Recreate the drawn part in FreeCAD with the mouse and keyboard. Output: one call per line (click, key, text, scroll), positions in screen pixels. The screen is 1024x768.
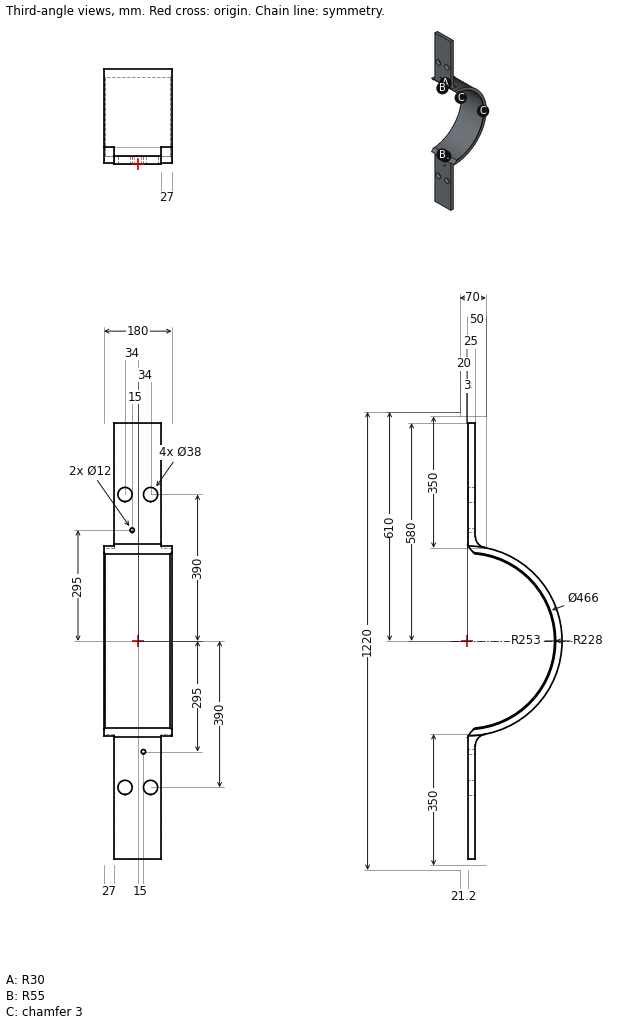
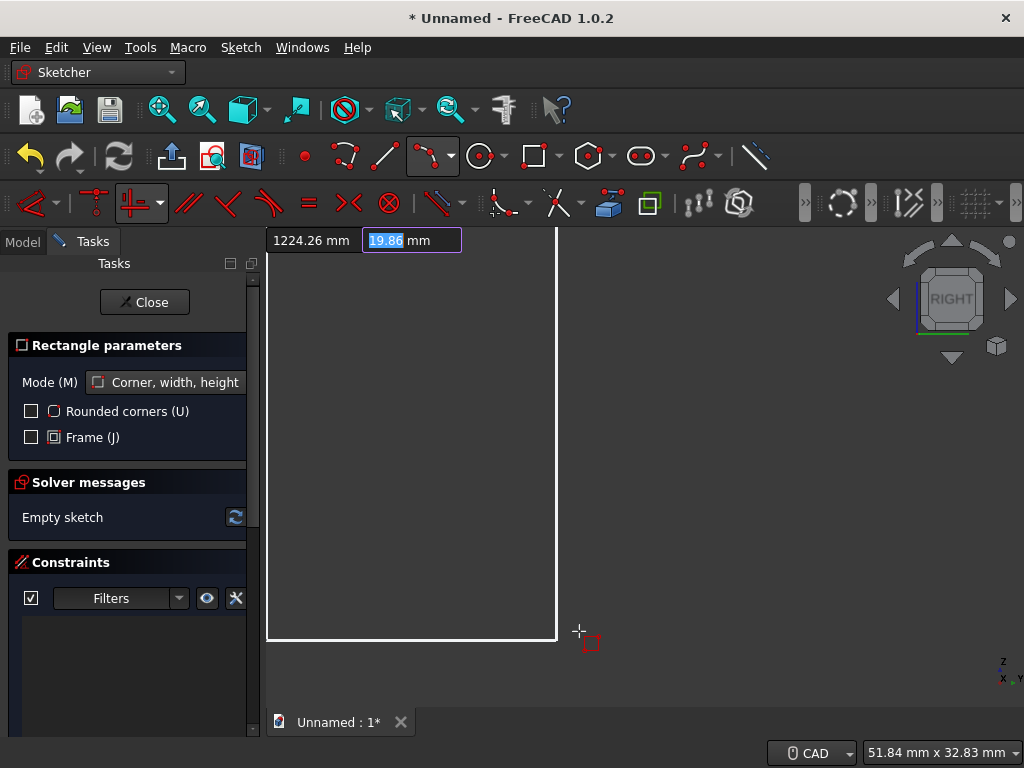
click(579, 561)
key(Escape)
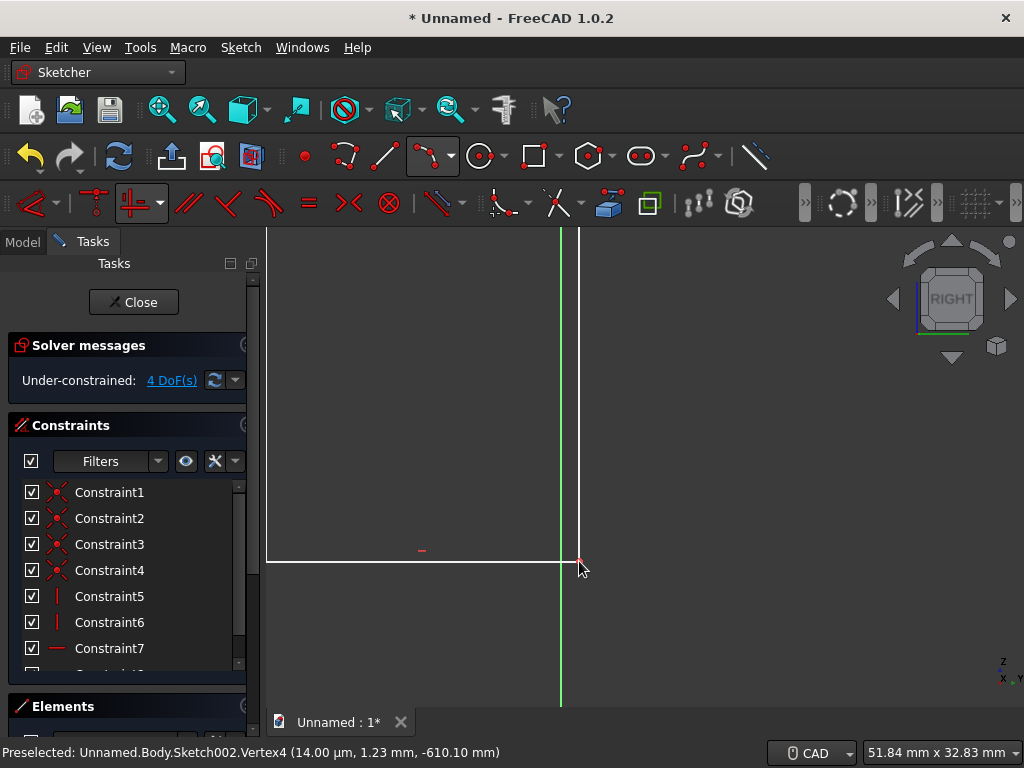
click(32, 204)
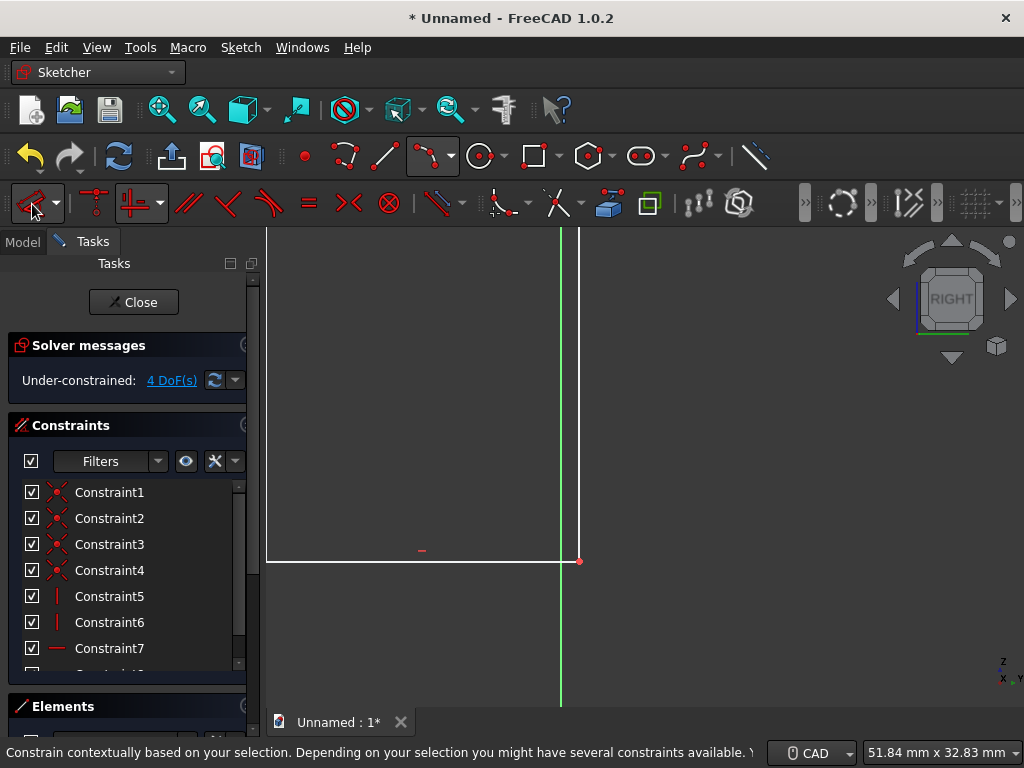
scroll(576, 467, down, 15)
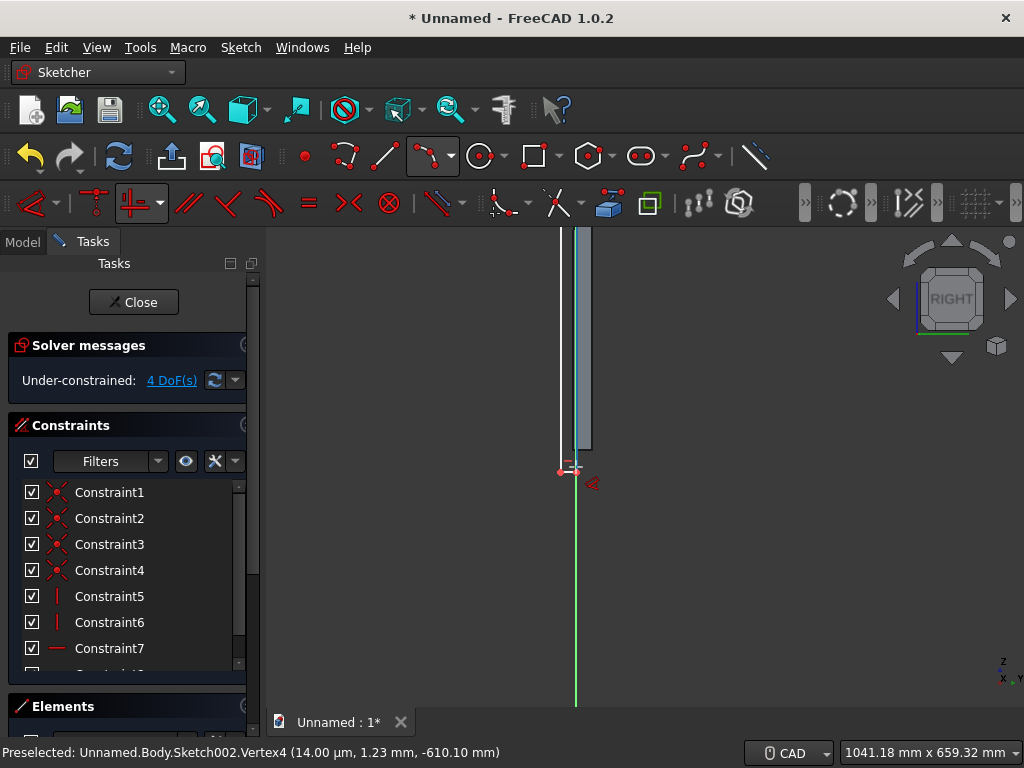
scroll(580, 656, down, 6)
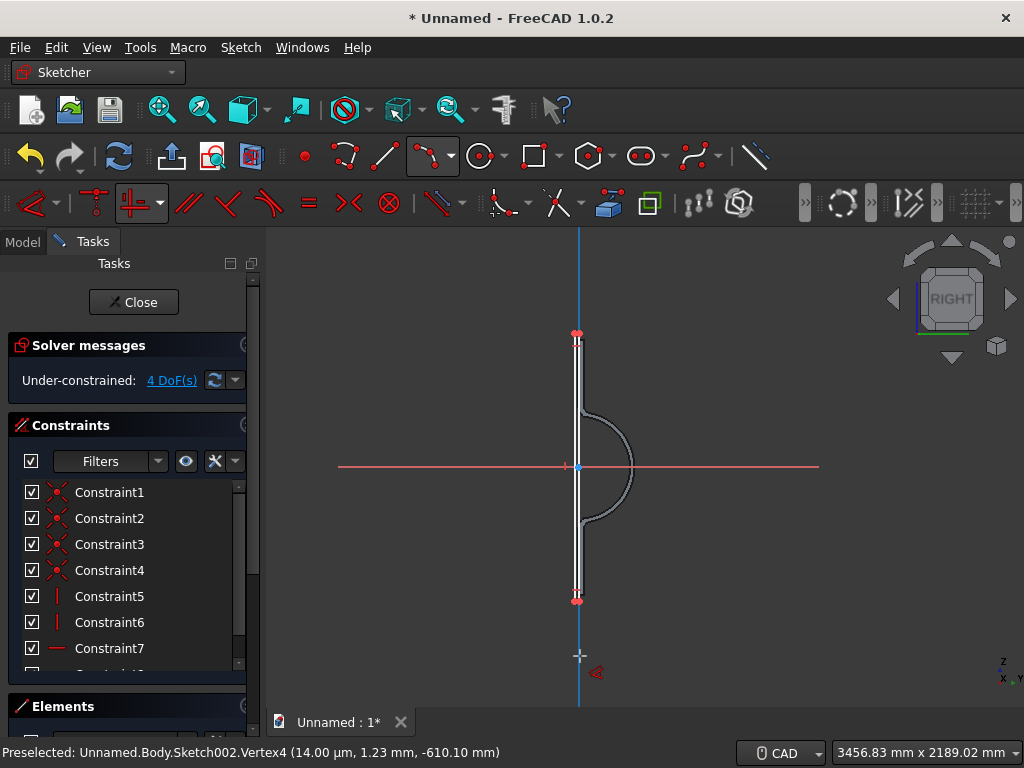
scroll(575, 334, up, 12)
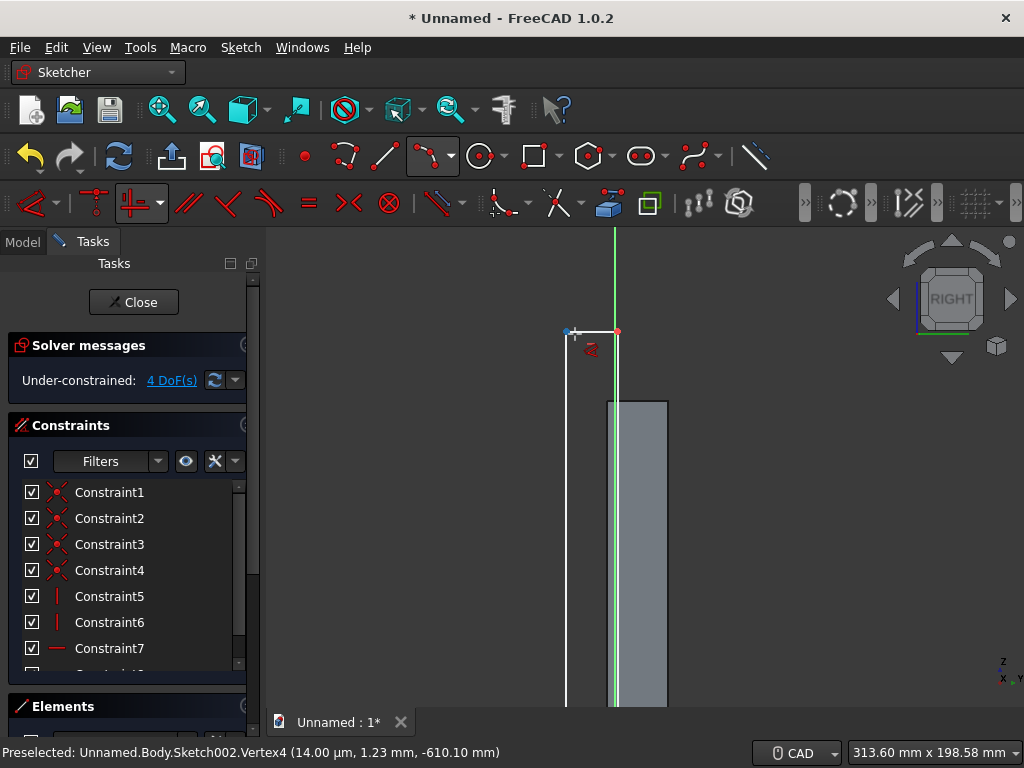
click(566, 332)
click(590, 298)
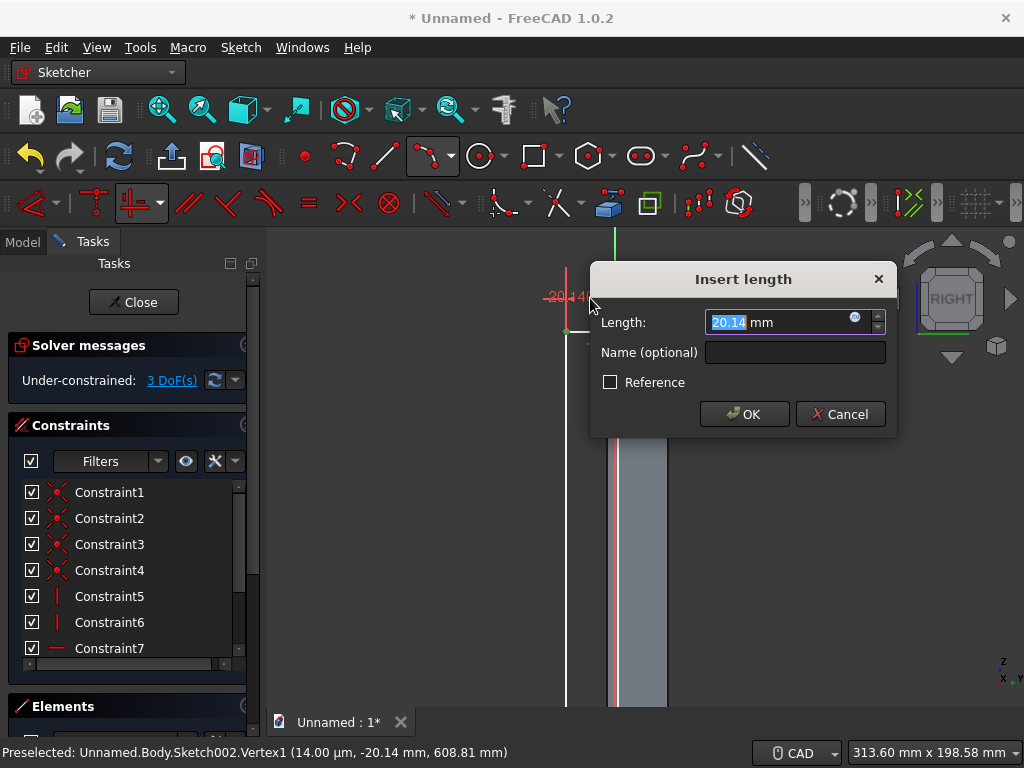
text(20)
key(Return)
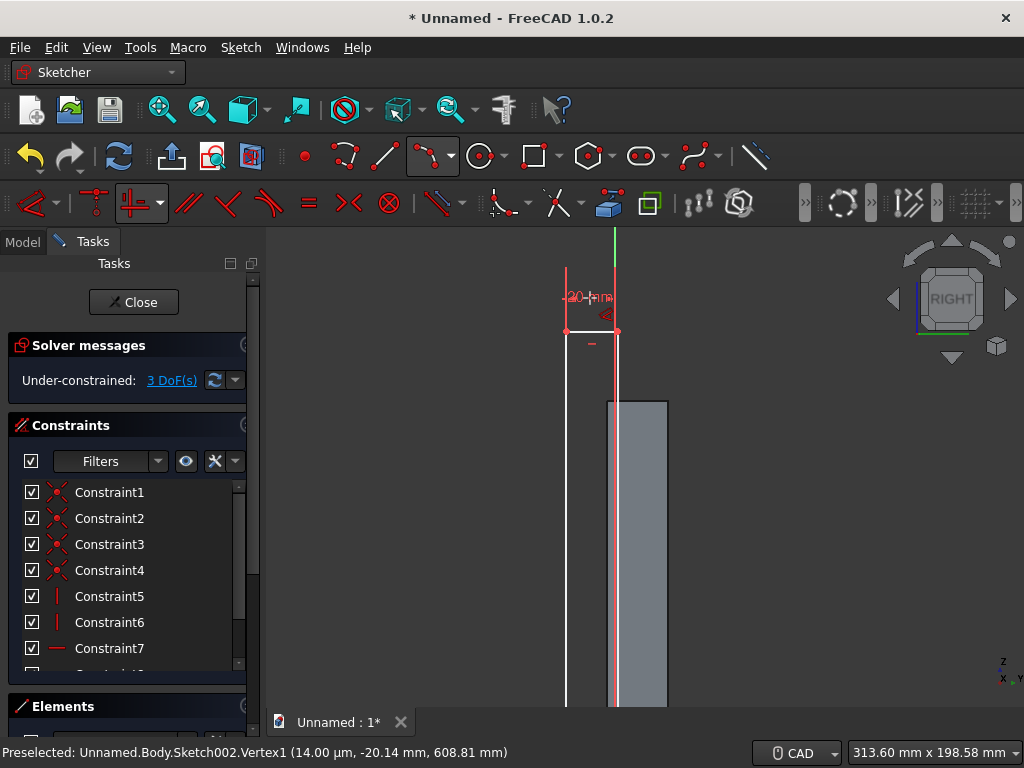
scroll(575, 300, down, 11)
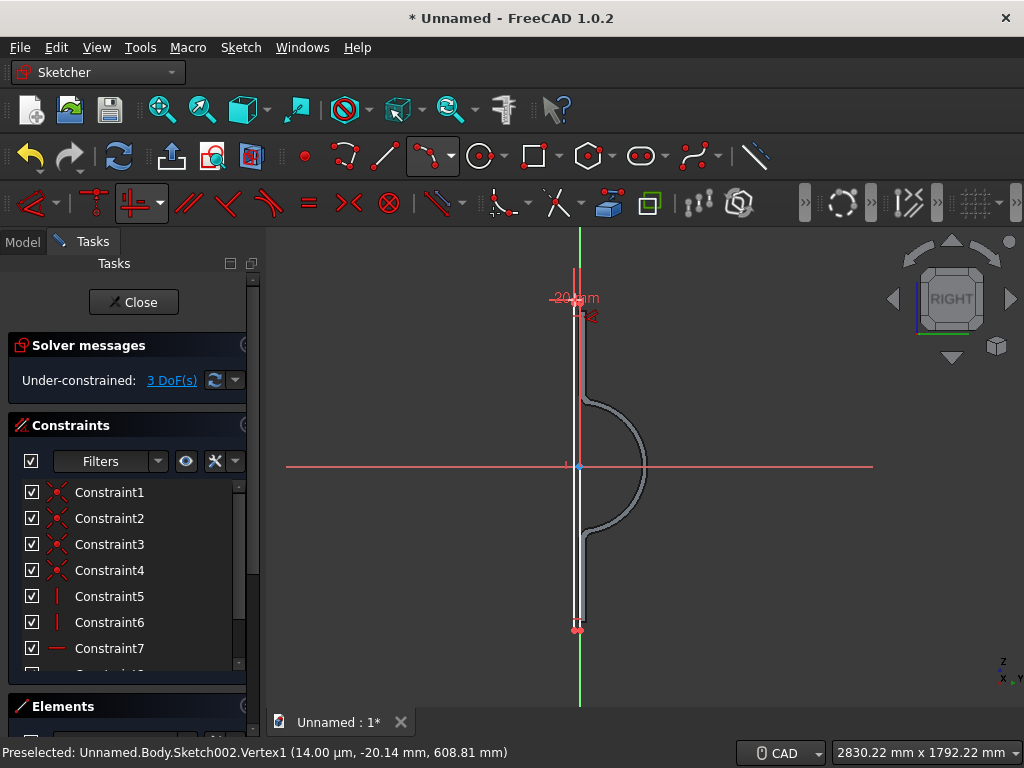
scroll(574, 402, up, 5)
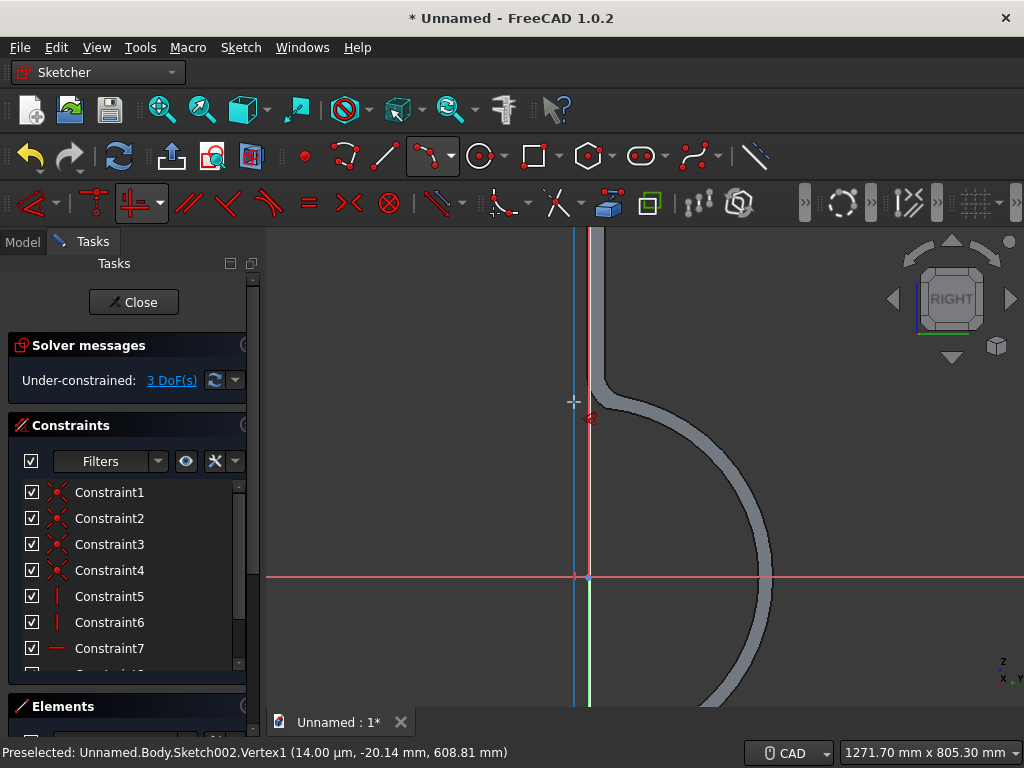
click(574, 400)
click(540, 467)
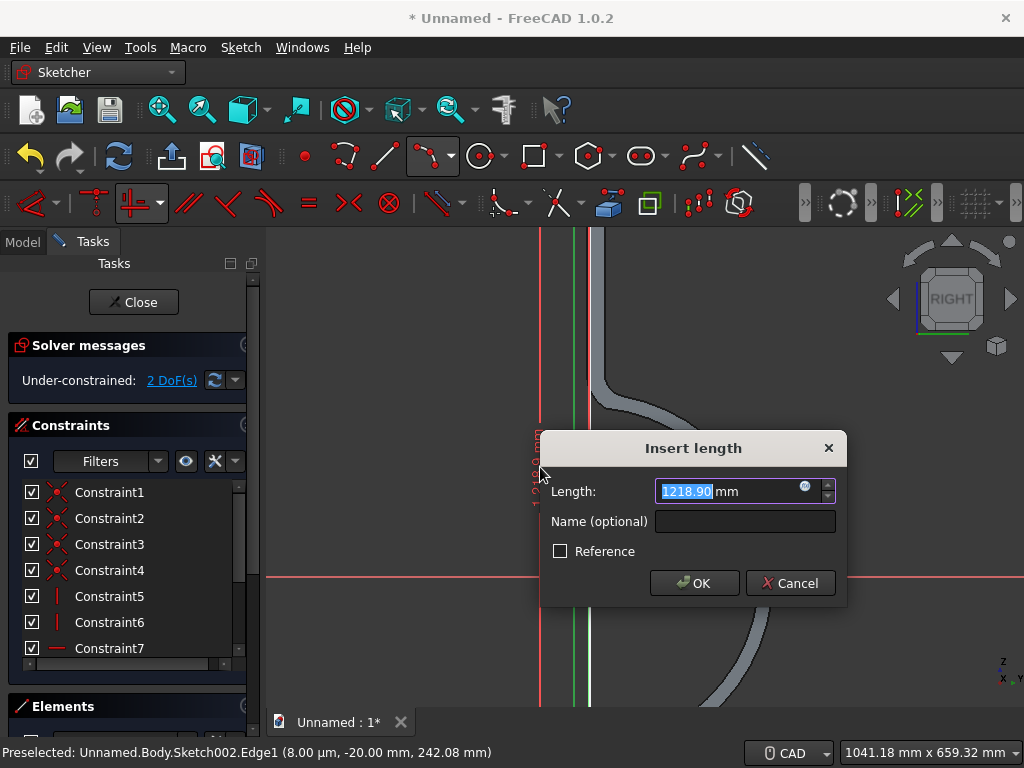
text(1220)
key(Return)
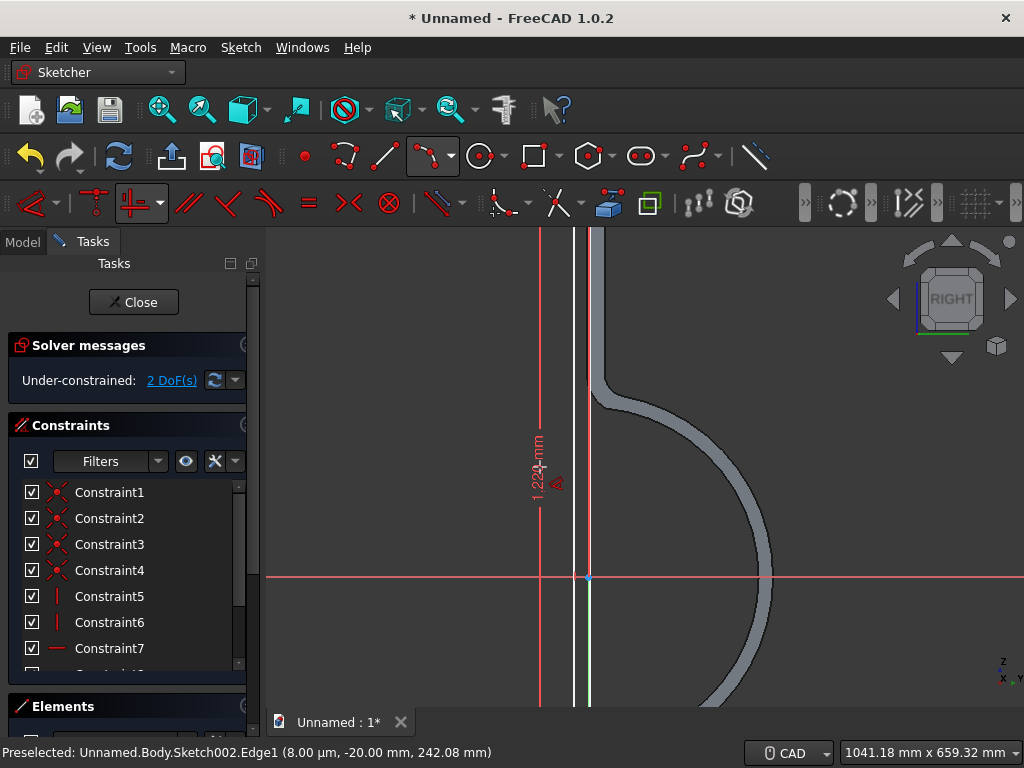
scroll(573, 403, down, 5)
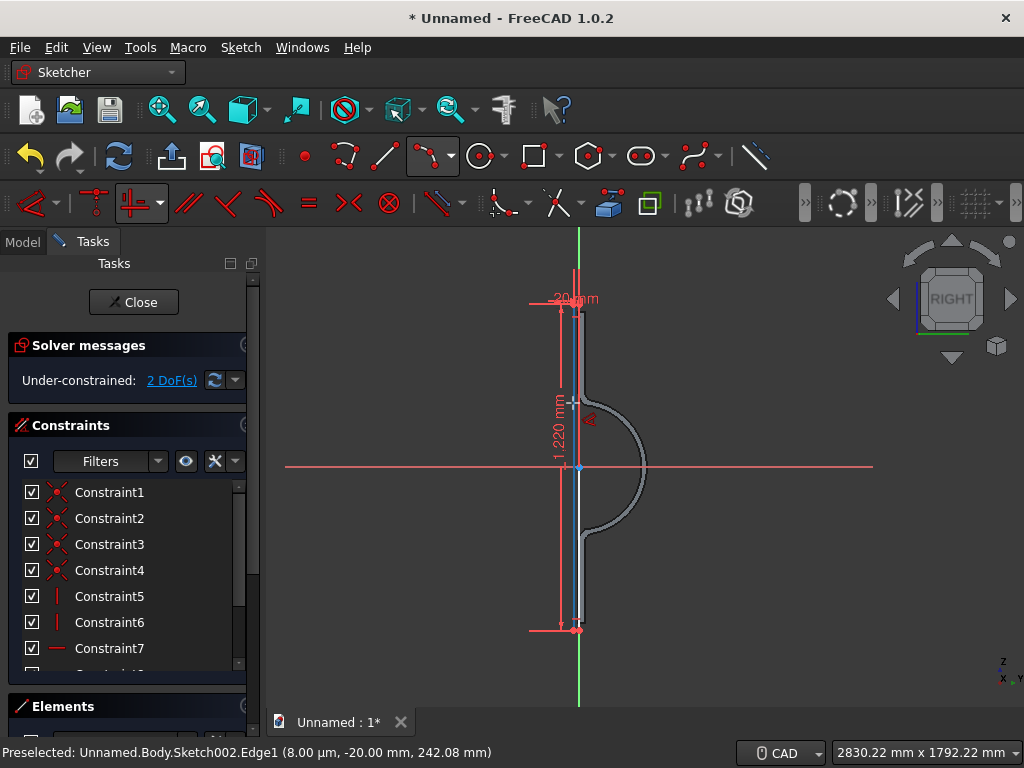
scroll(577, 631, up, 10)